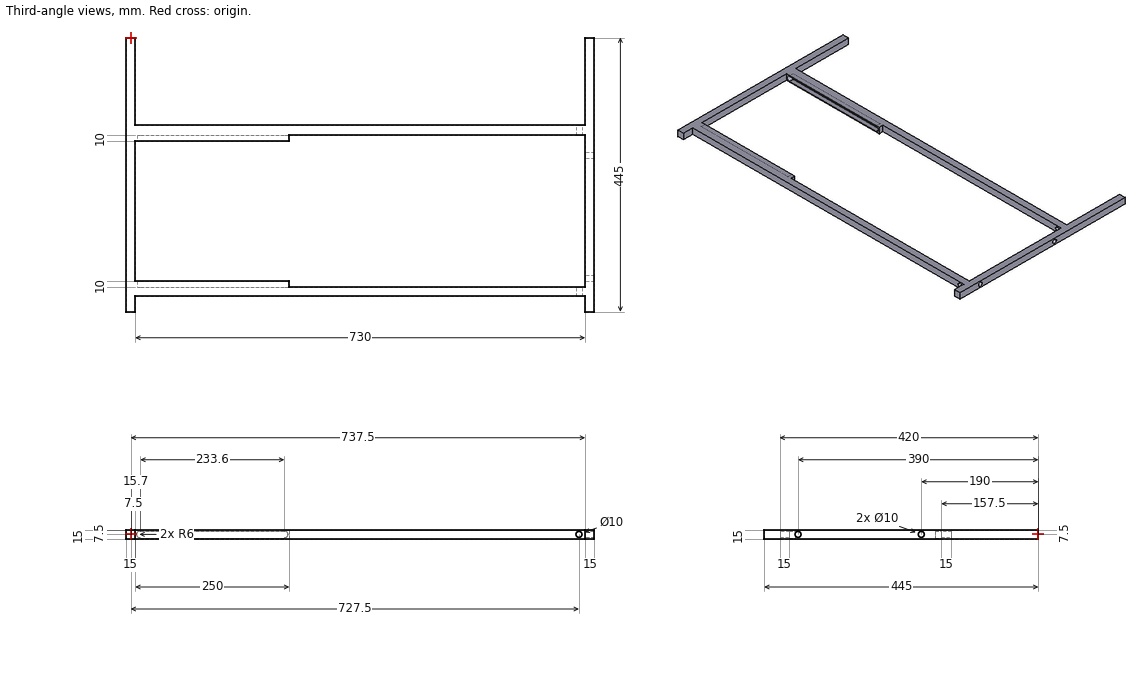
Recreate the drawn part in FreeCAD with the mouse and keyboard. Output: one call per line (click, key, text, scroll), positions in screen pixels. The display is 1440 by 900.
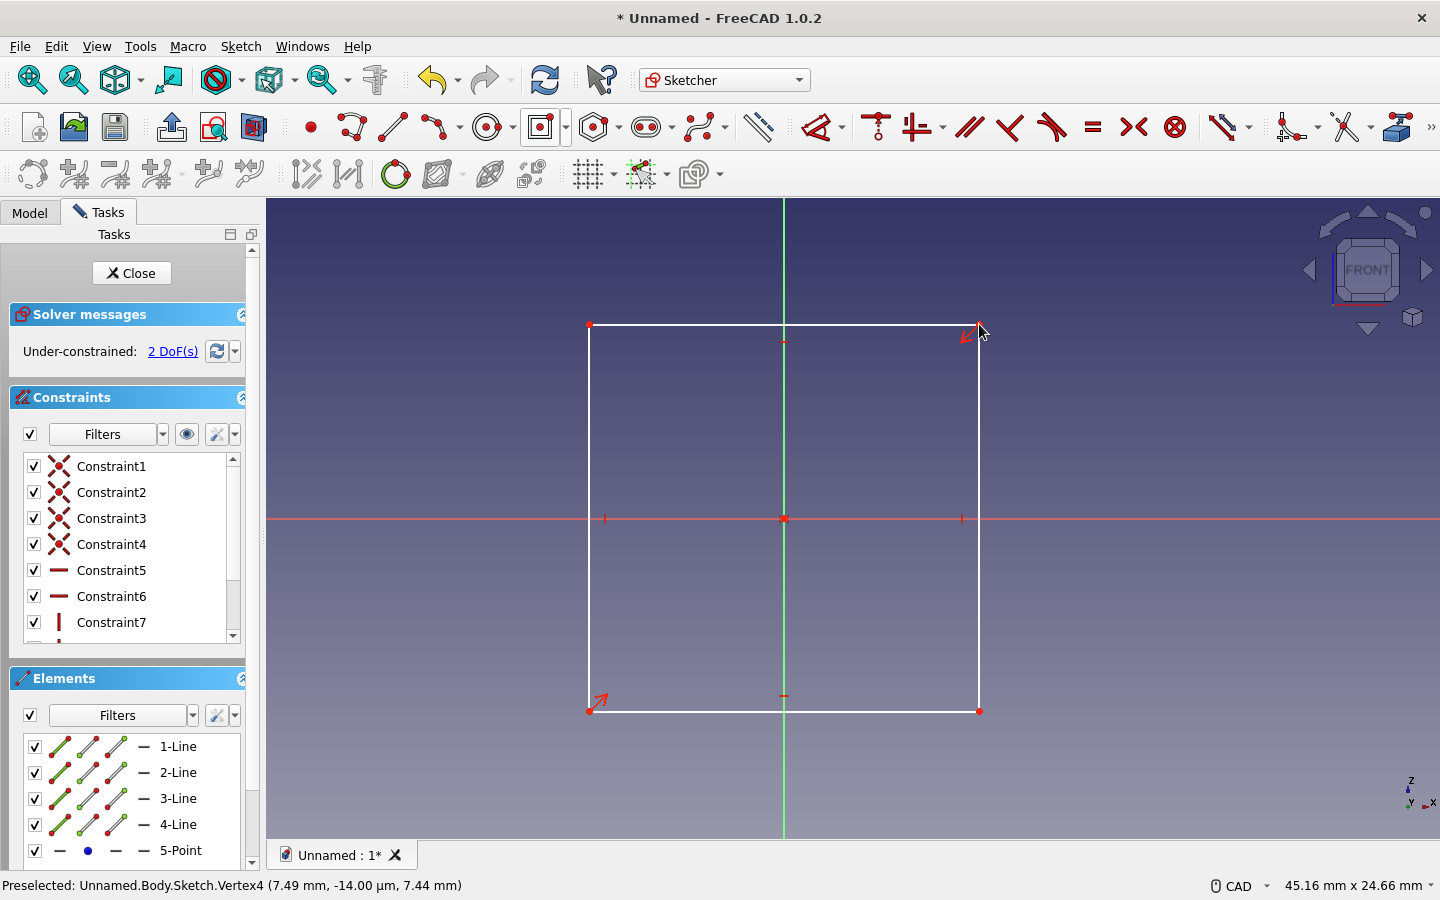
click(816, 128)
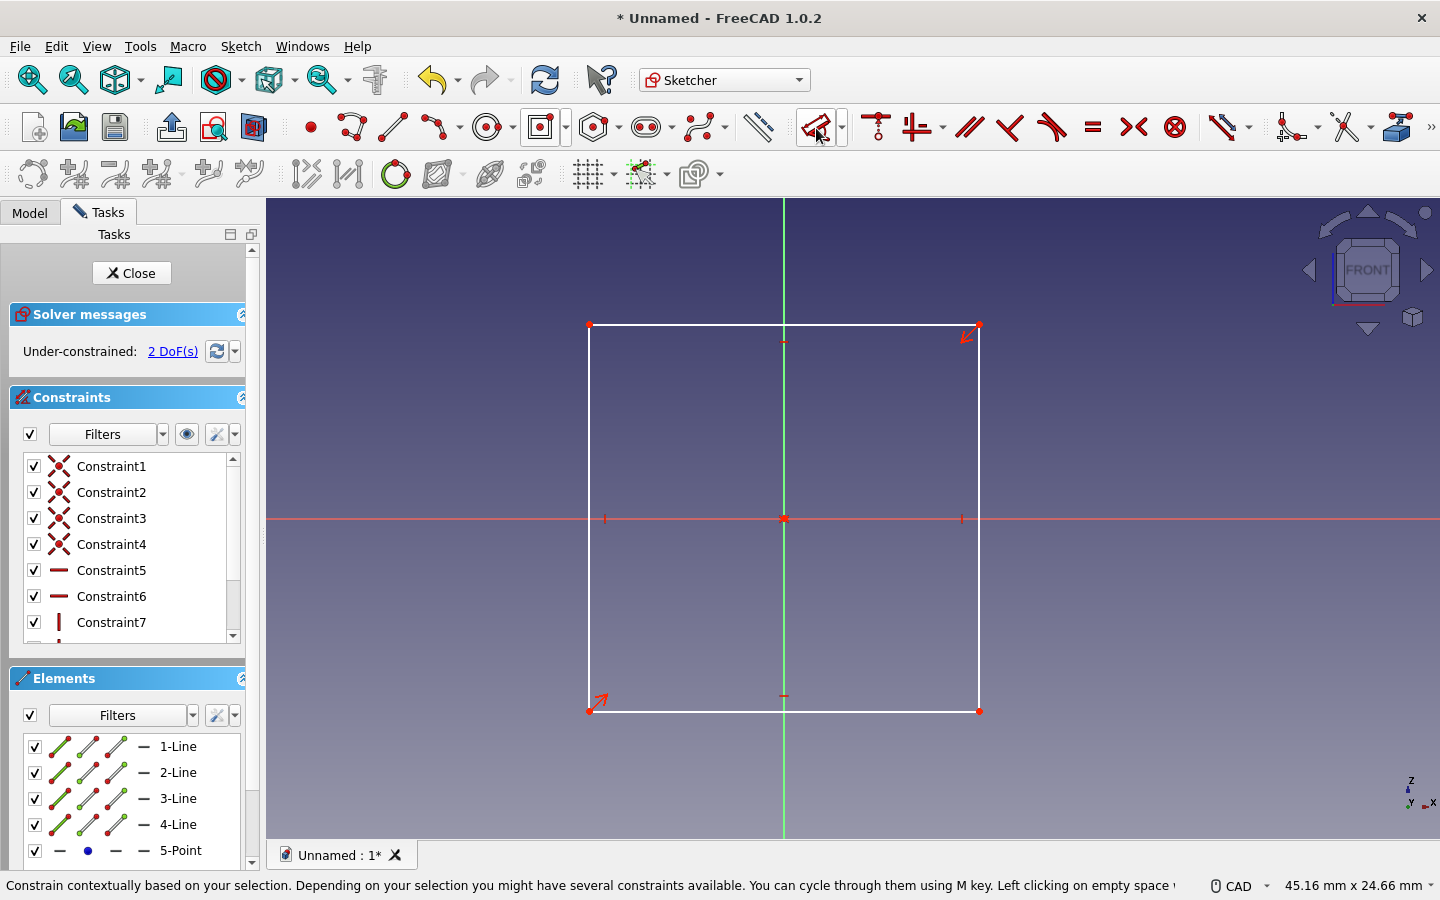
click(706, 712)
click(695, 746)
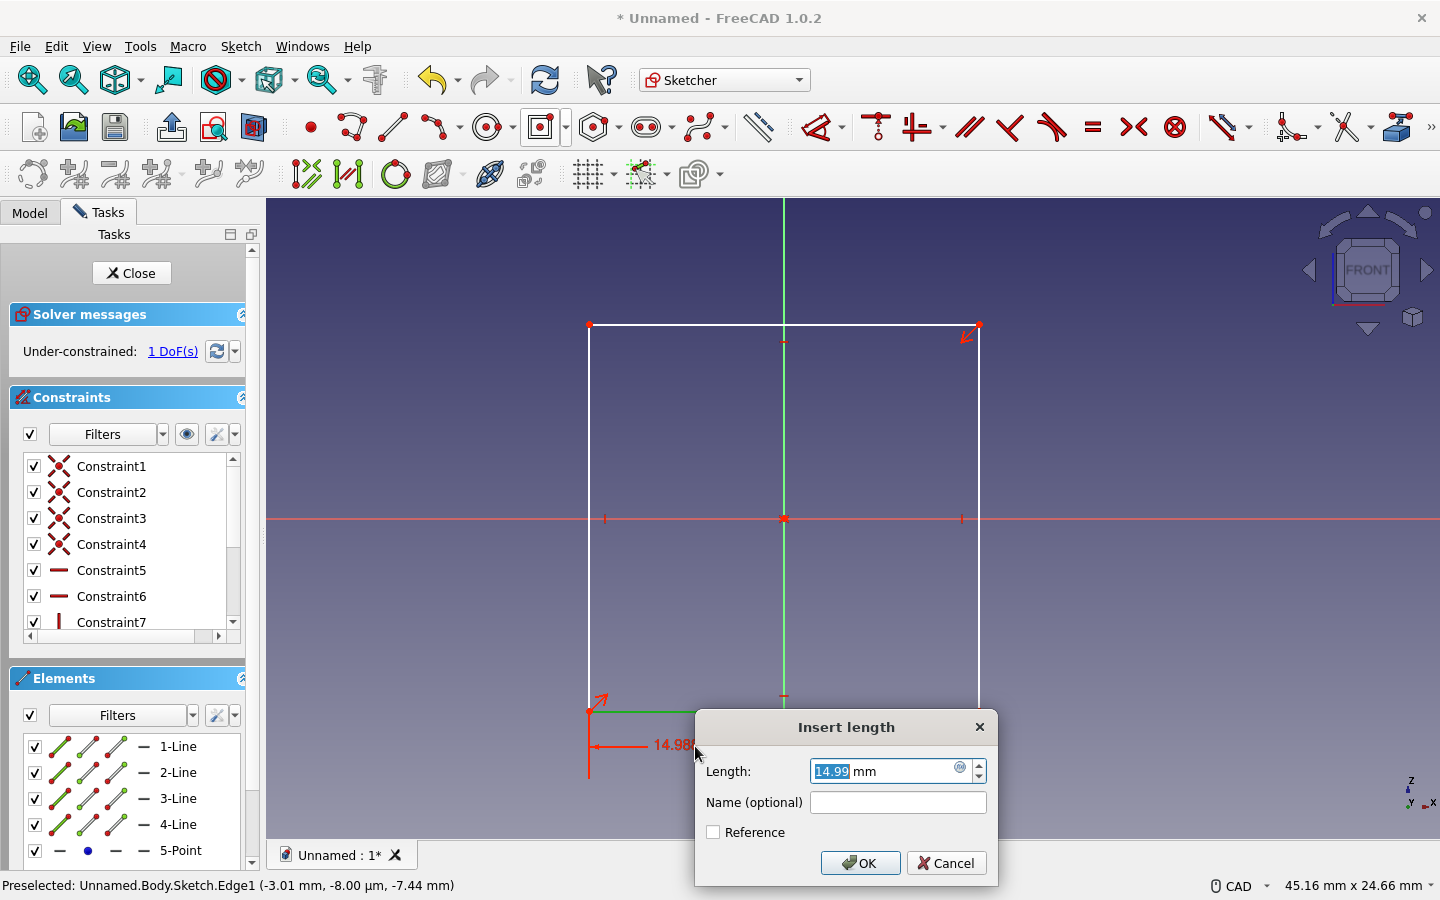
text(15)
key(Return)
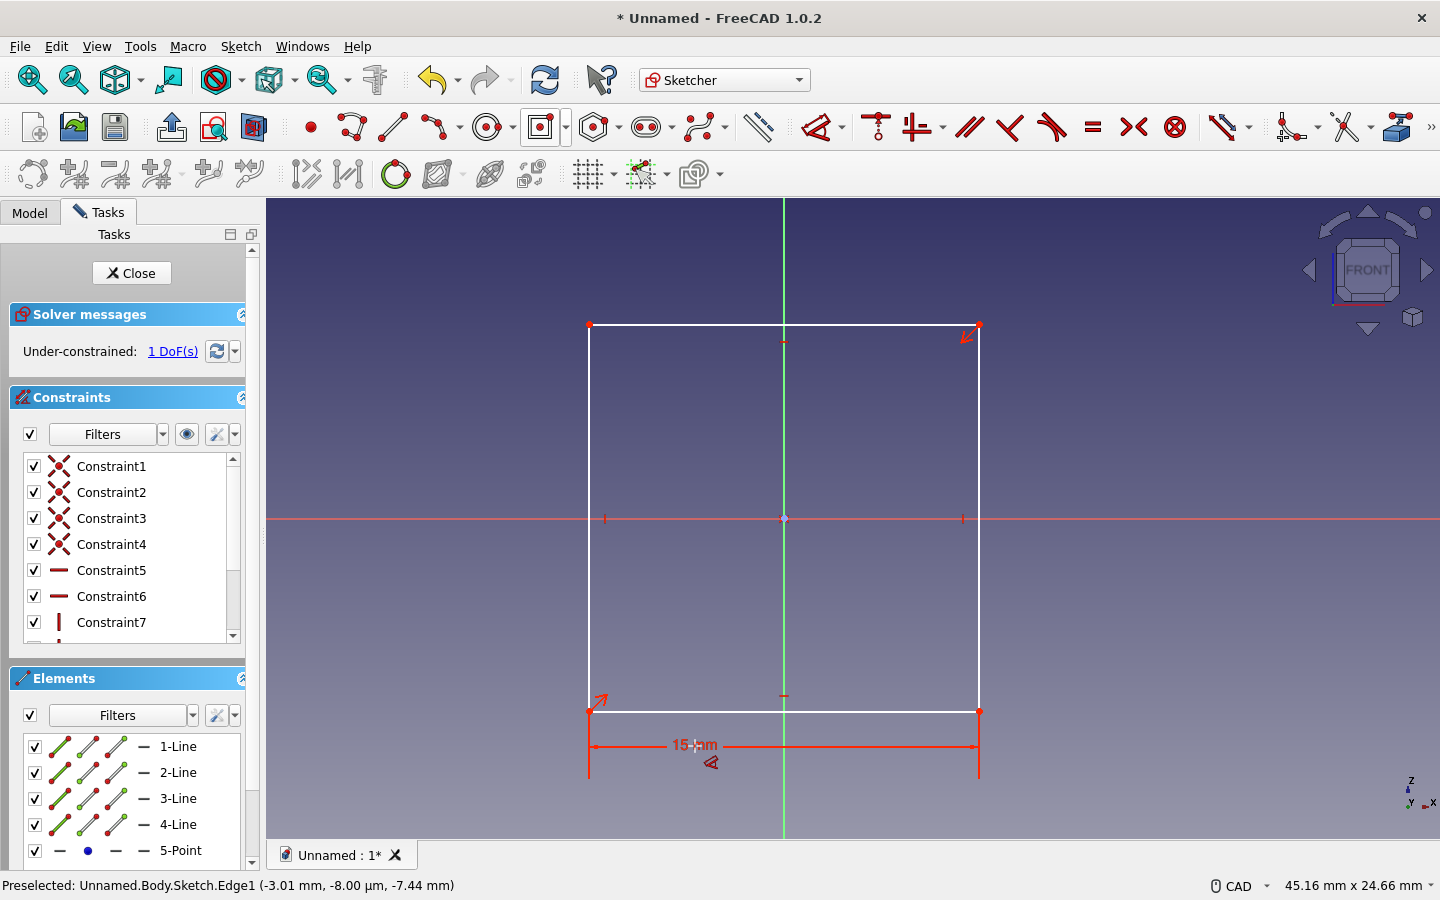
click(979, 596)
click(1013, 429)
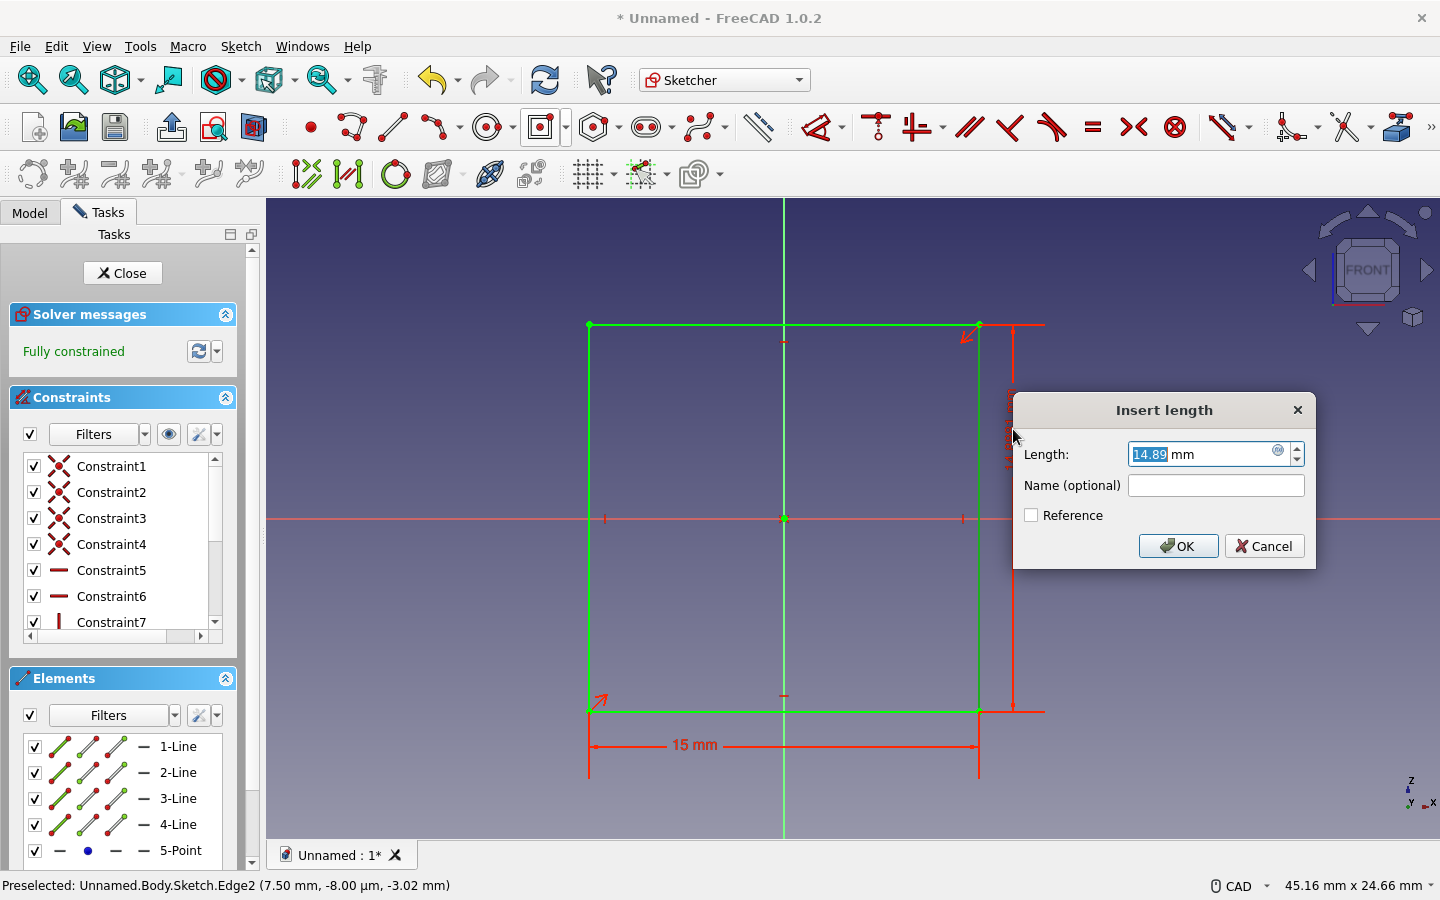
text(15)
key(Return)
key(Escape)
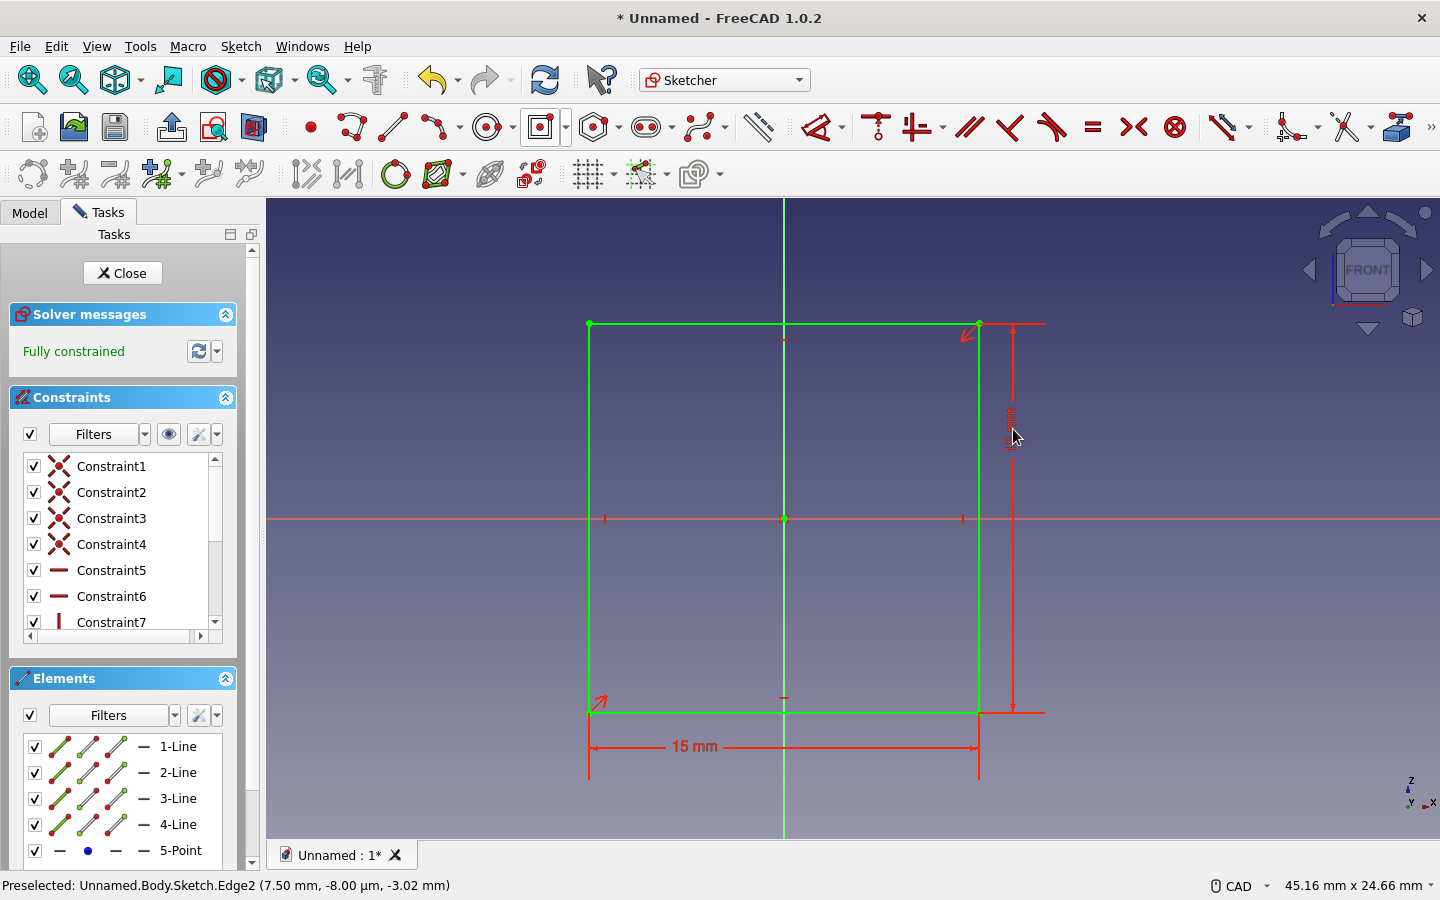
click(123, 273)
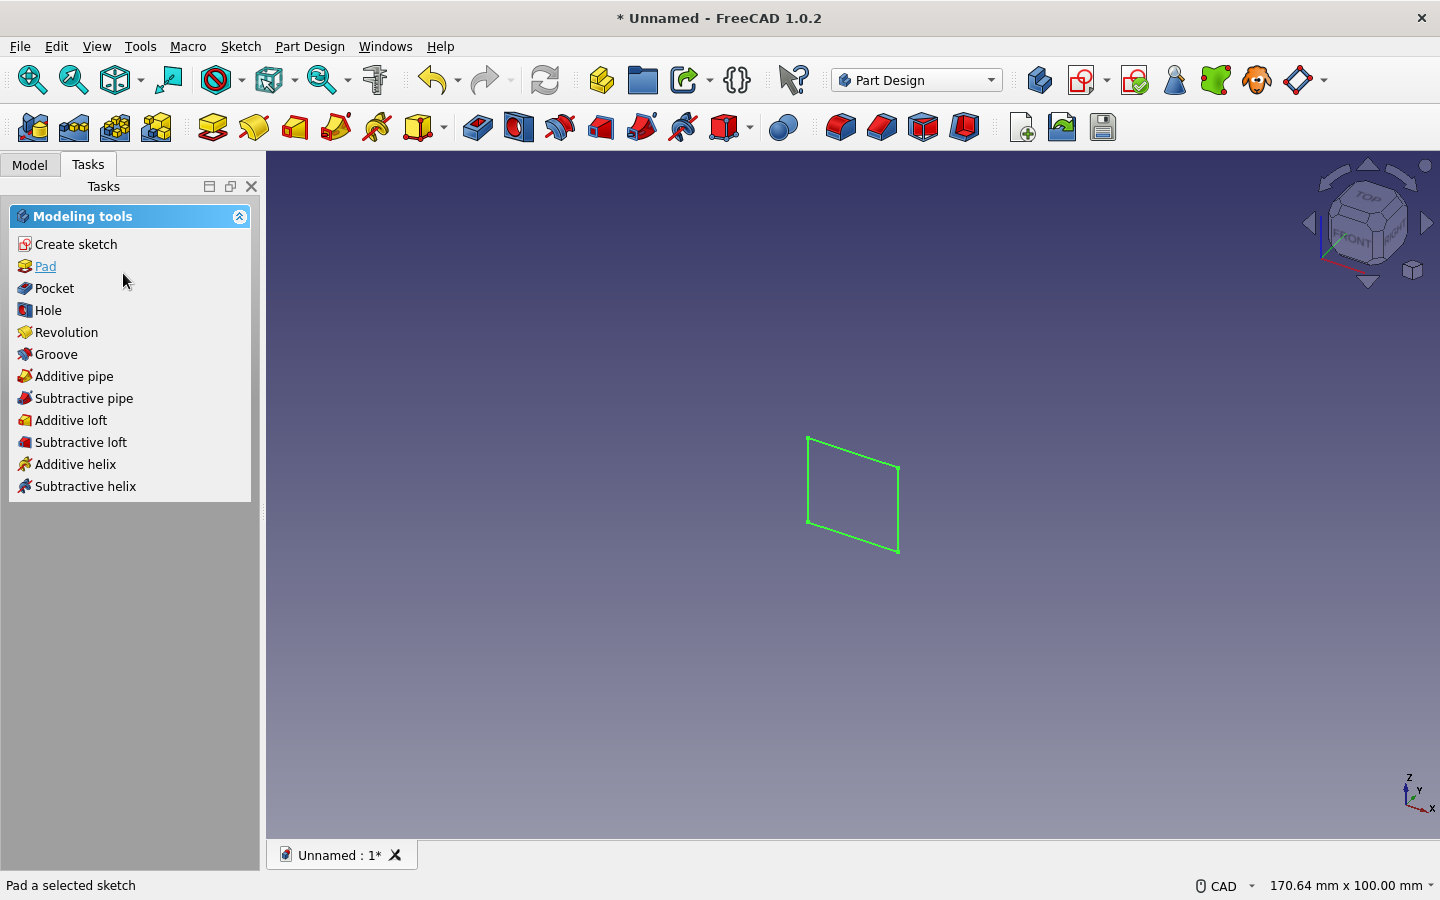
click(213, 128)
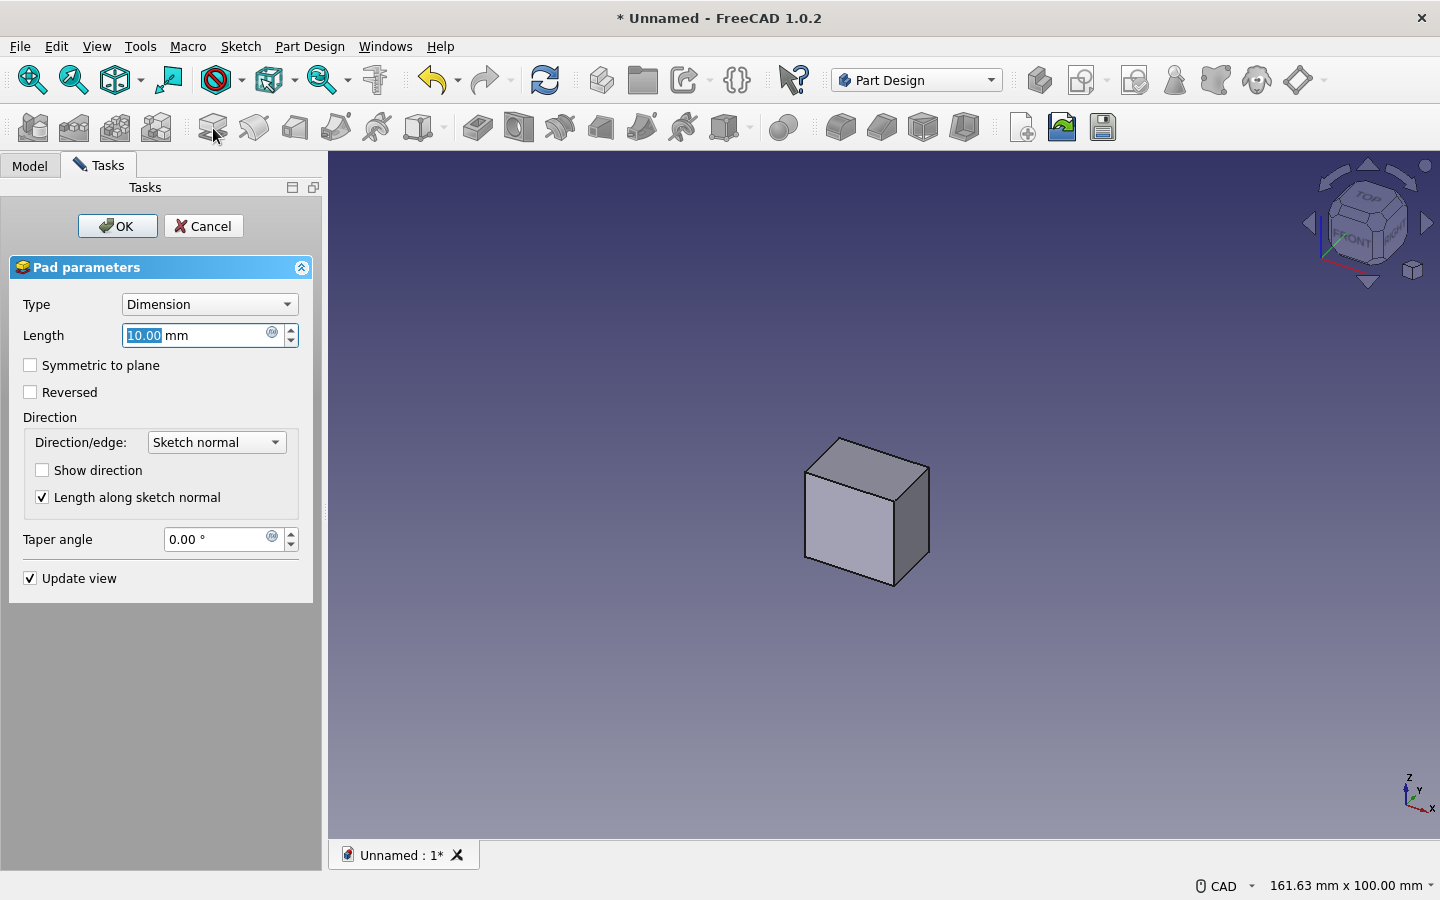
text(445)
key(Tab)